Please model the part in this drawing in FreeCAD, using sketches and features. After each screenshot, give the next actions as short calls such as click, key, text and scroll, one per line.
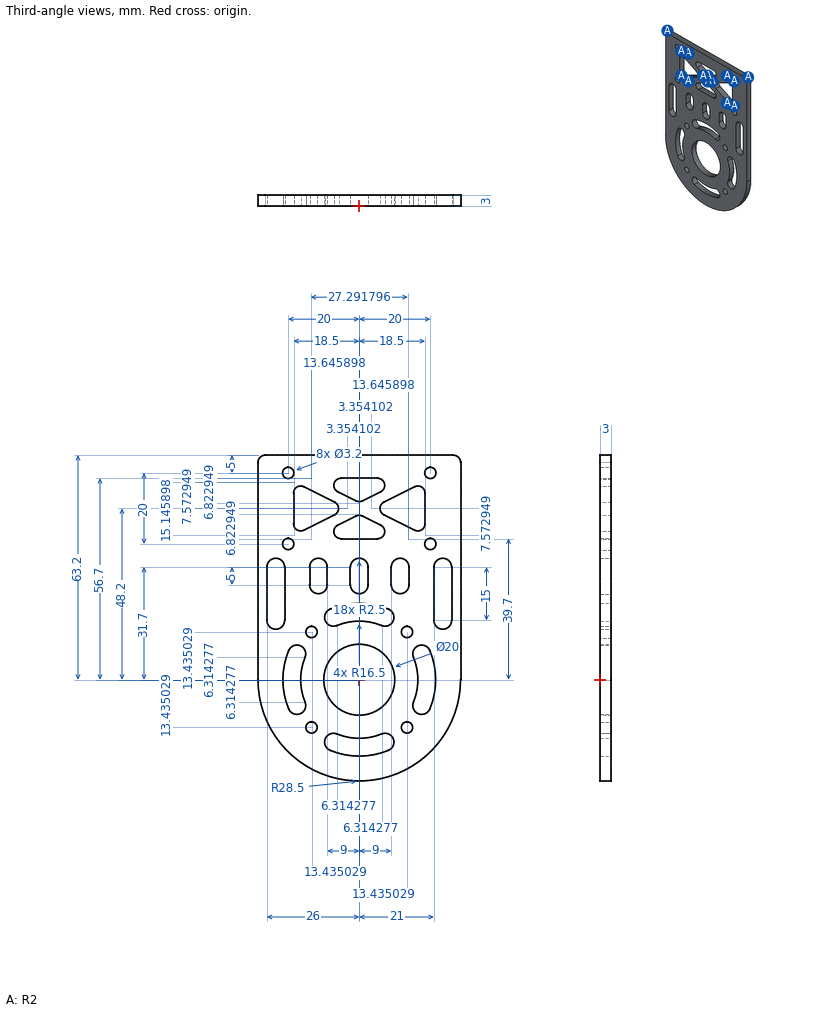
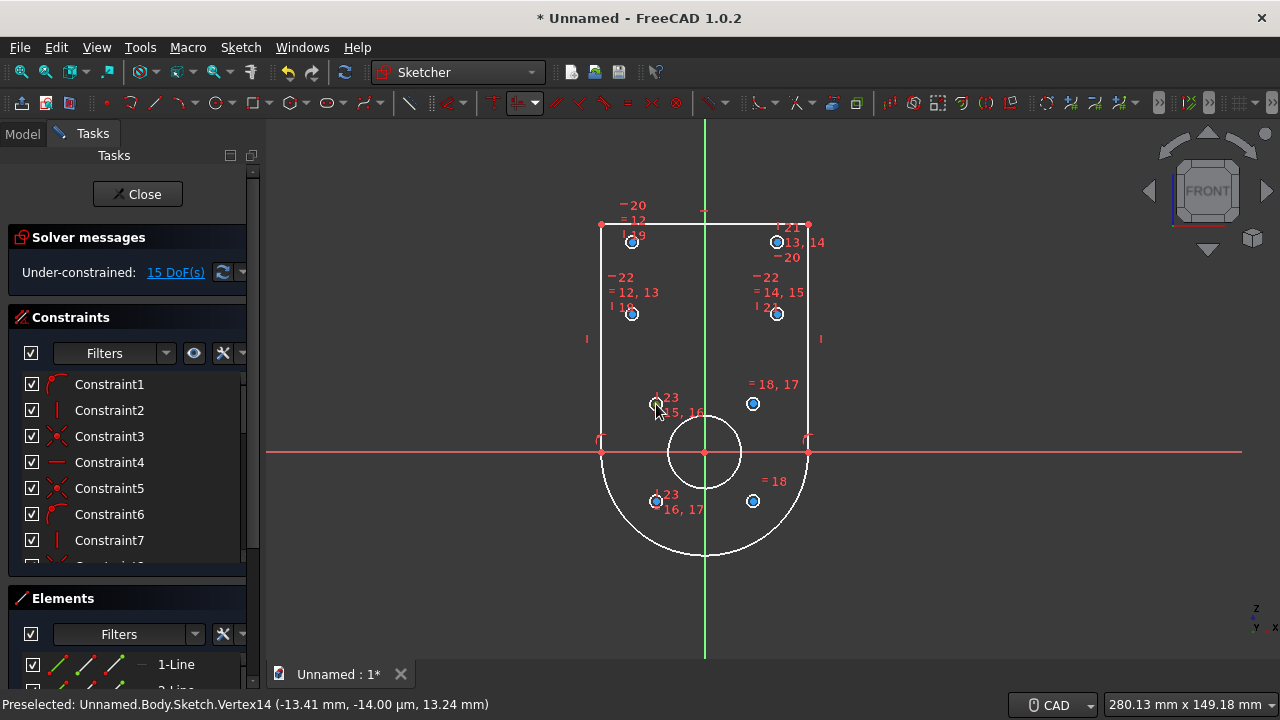
click(753, 404)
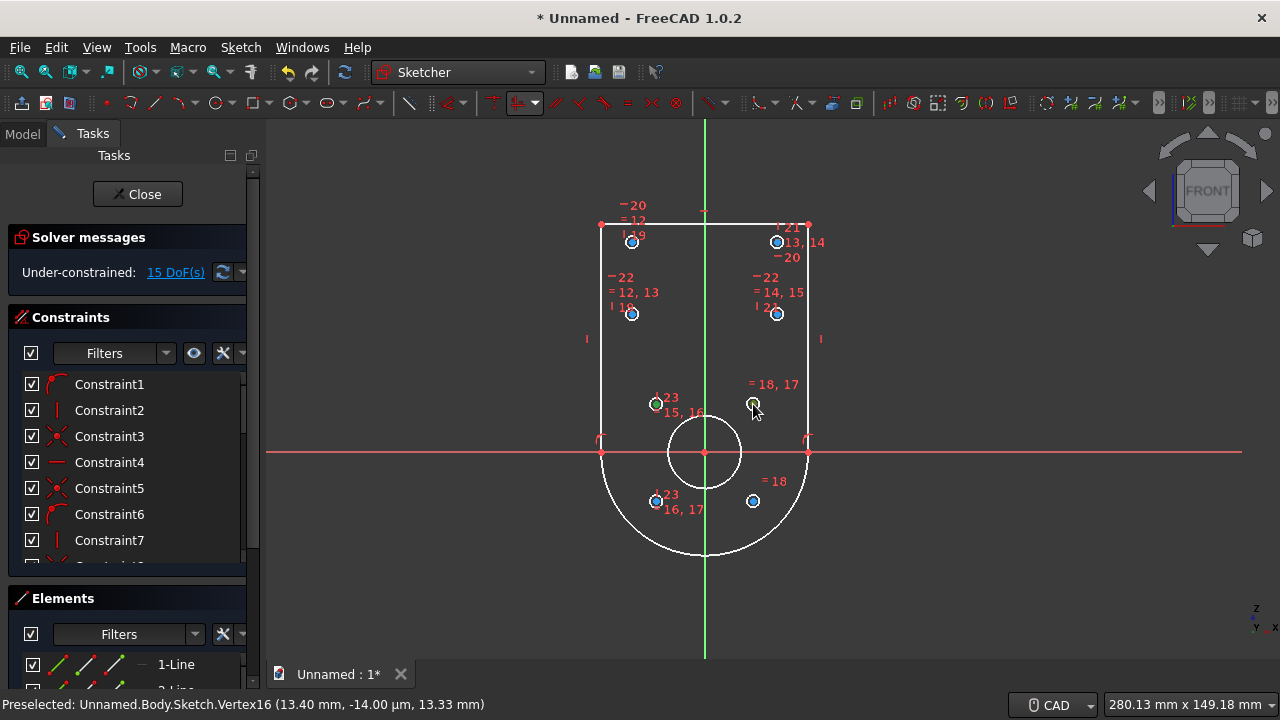
key(h)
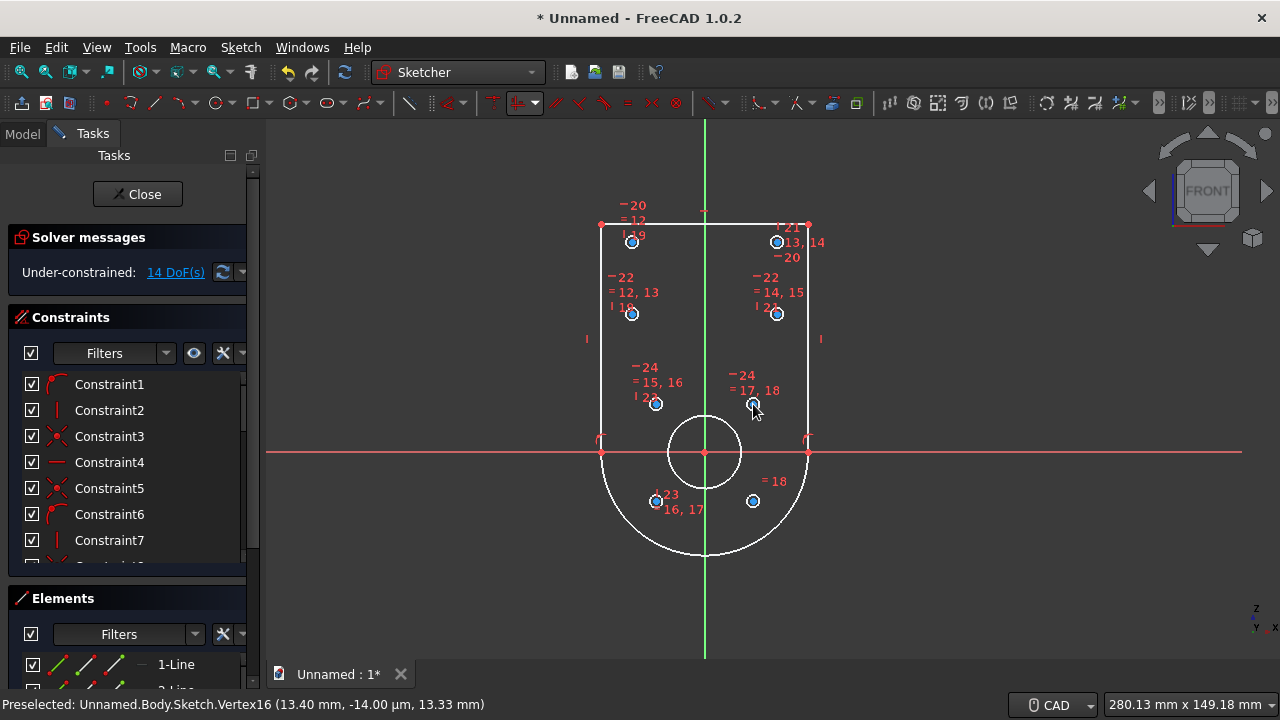
click(753, 404)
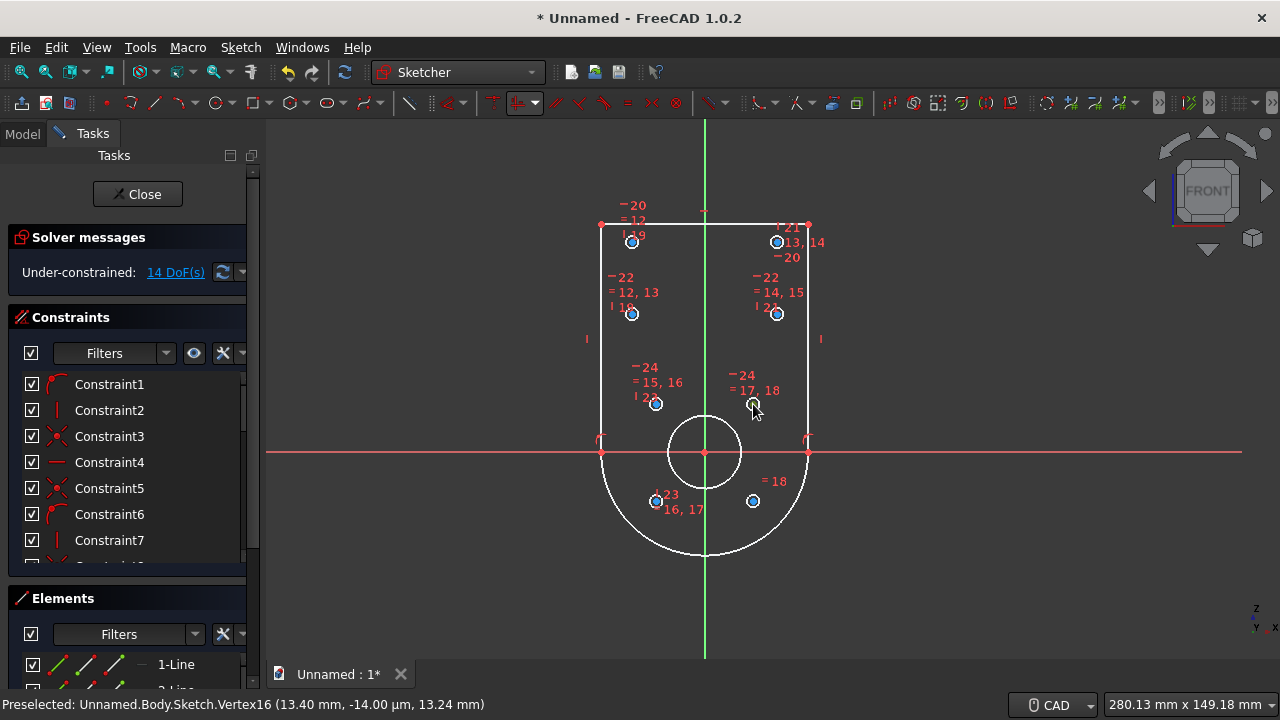
click(753, 501)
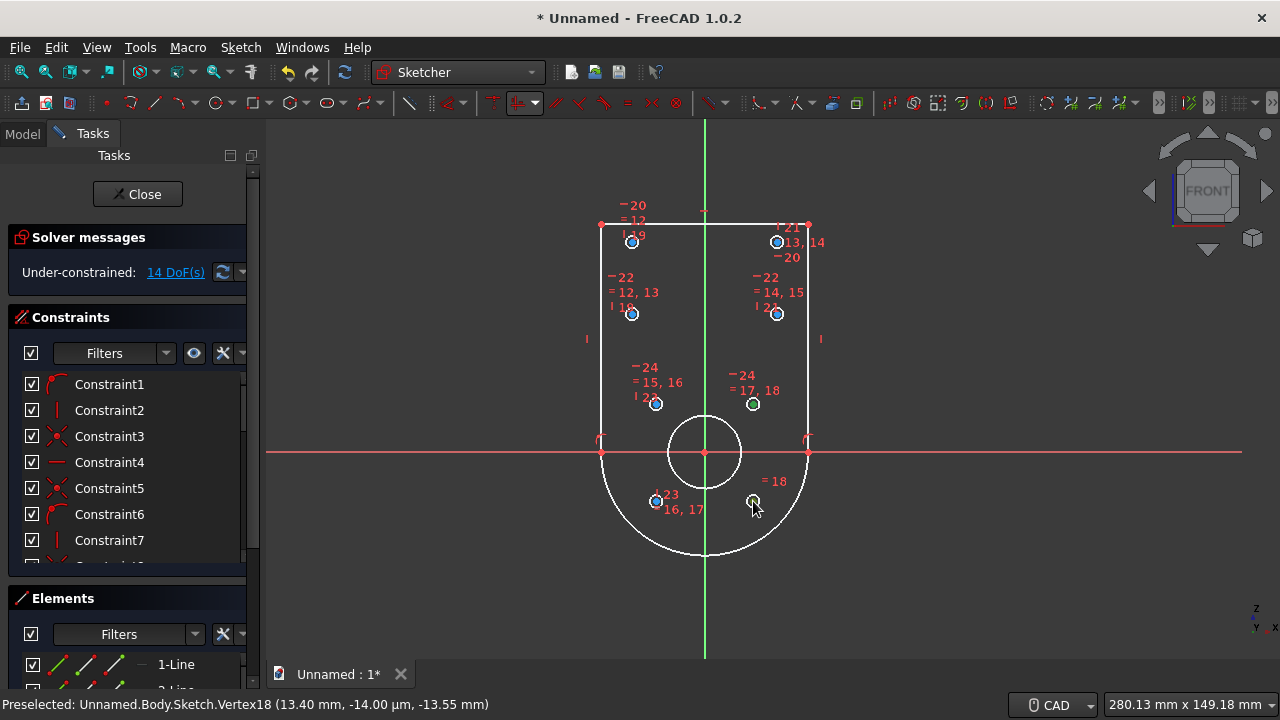
key(v)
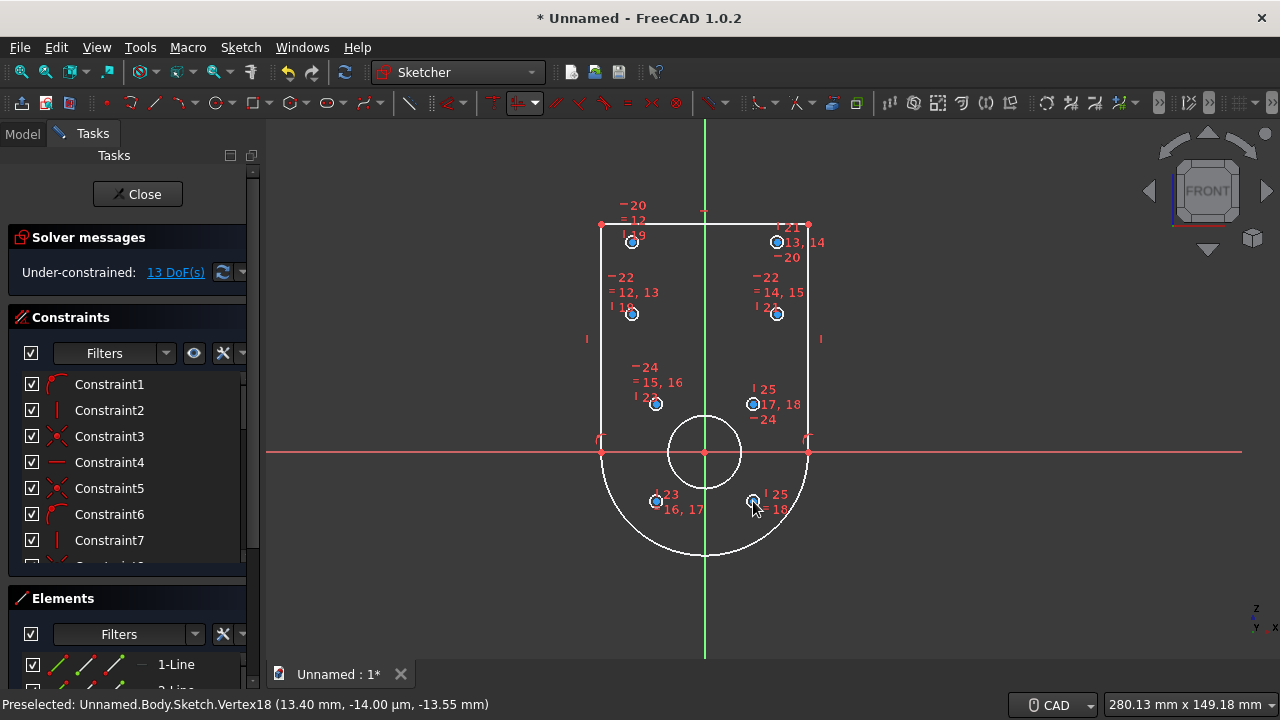
scroll(656, 501, up, 4)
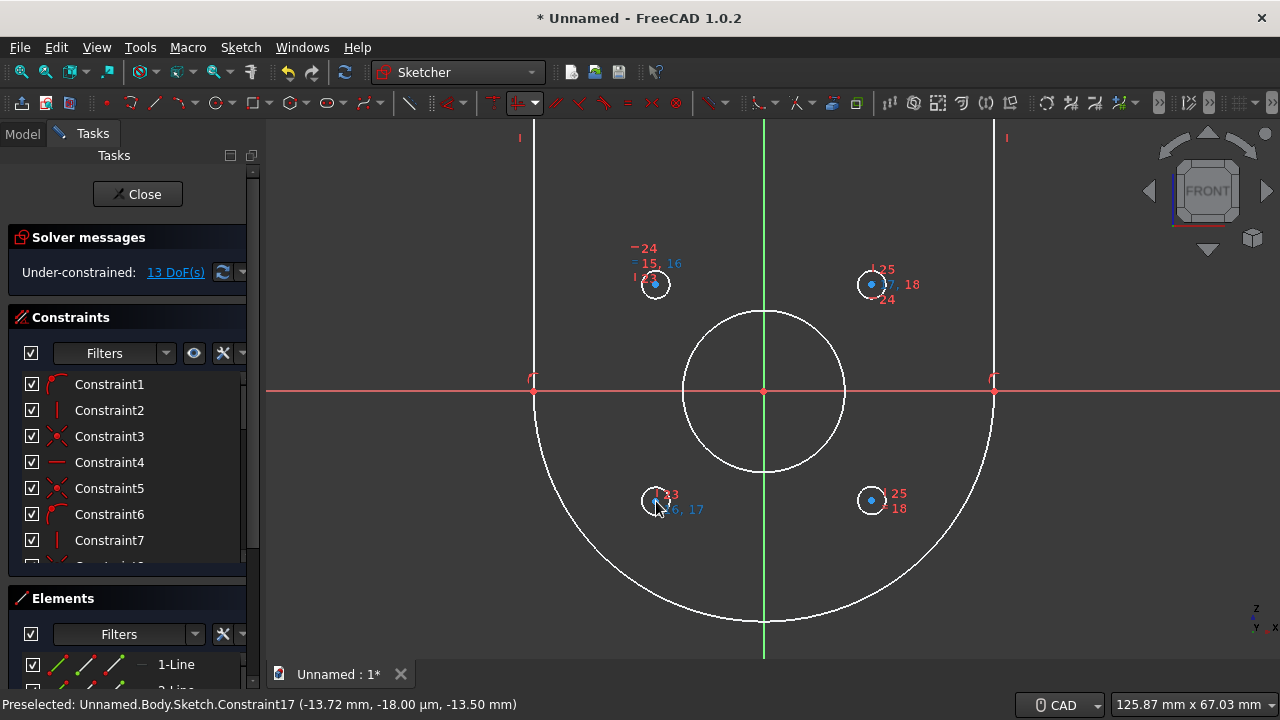
scroll(656, 501, up, 4)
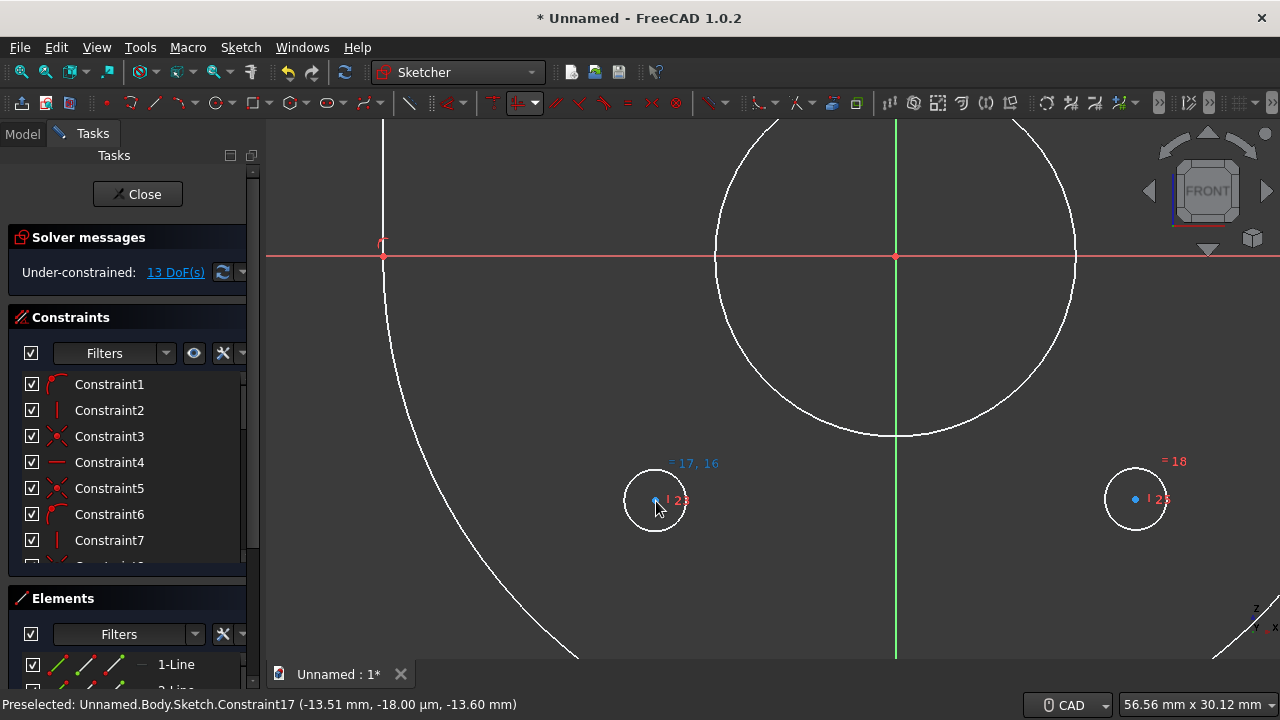
click(655, 501)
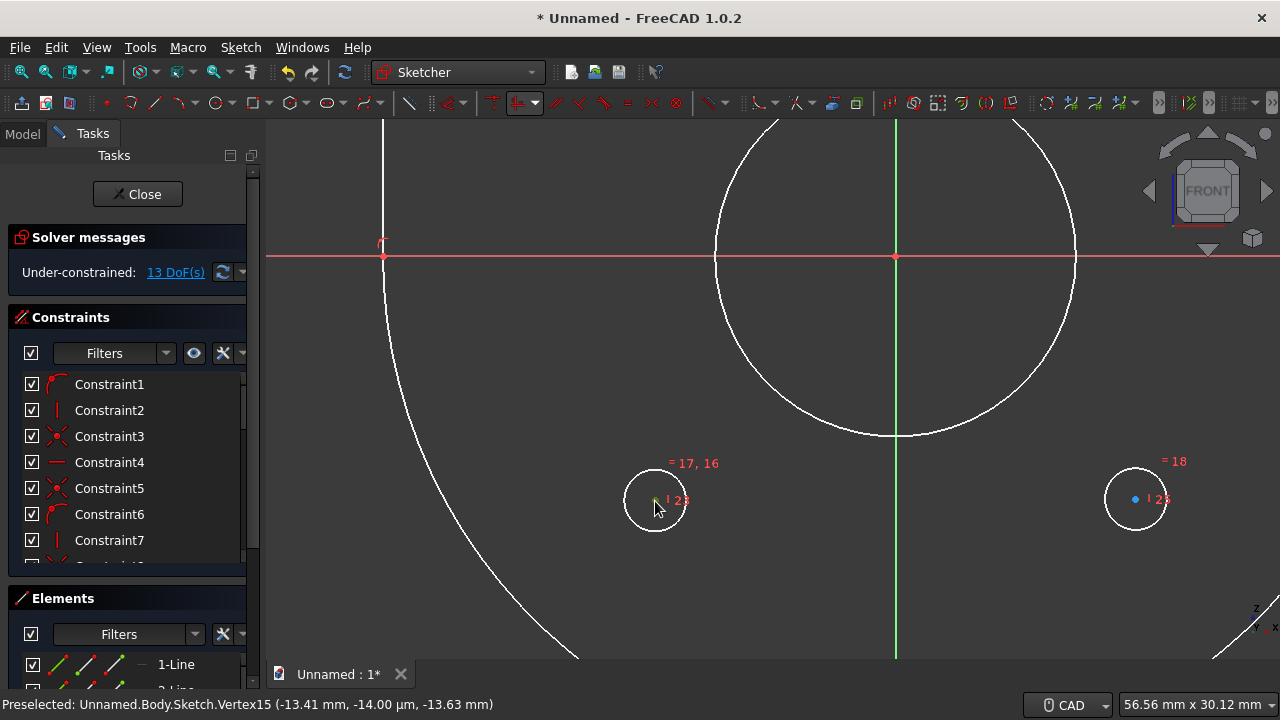
scroll(656, 501, down, 8)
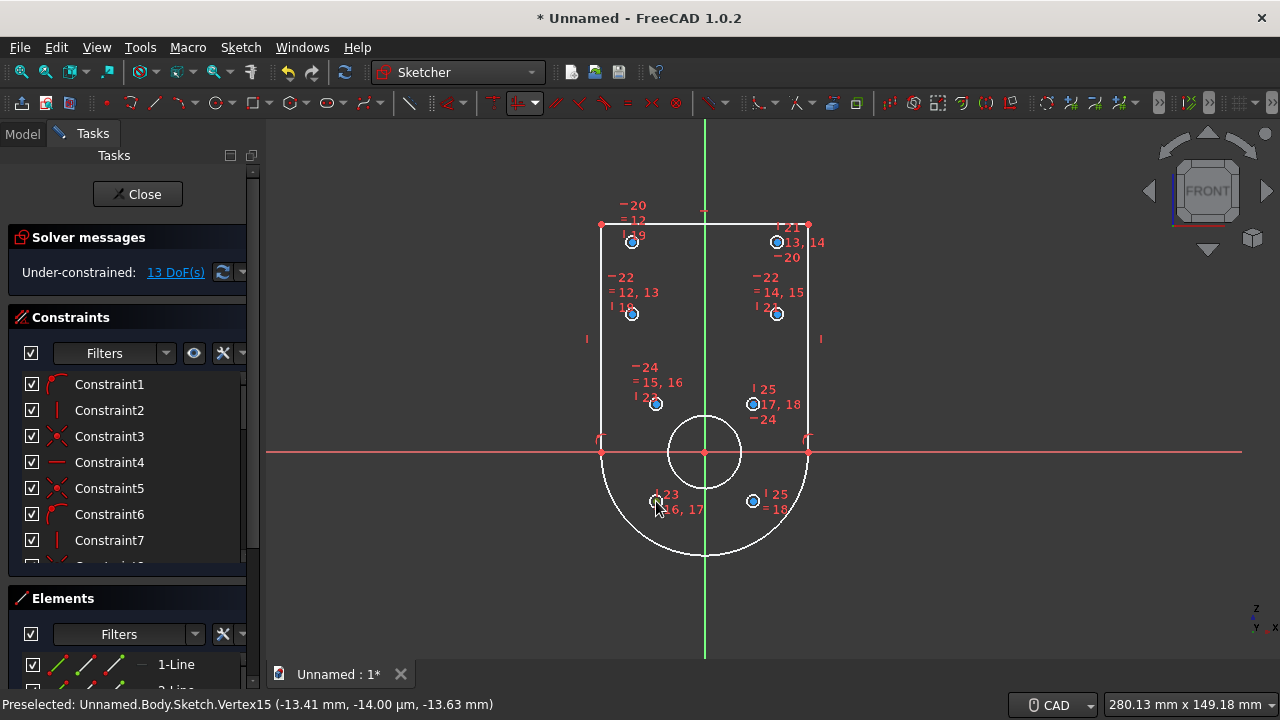
click(753, 501)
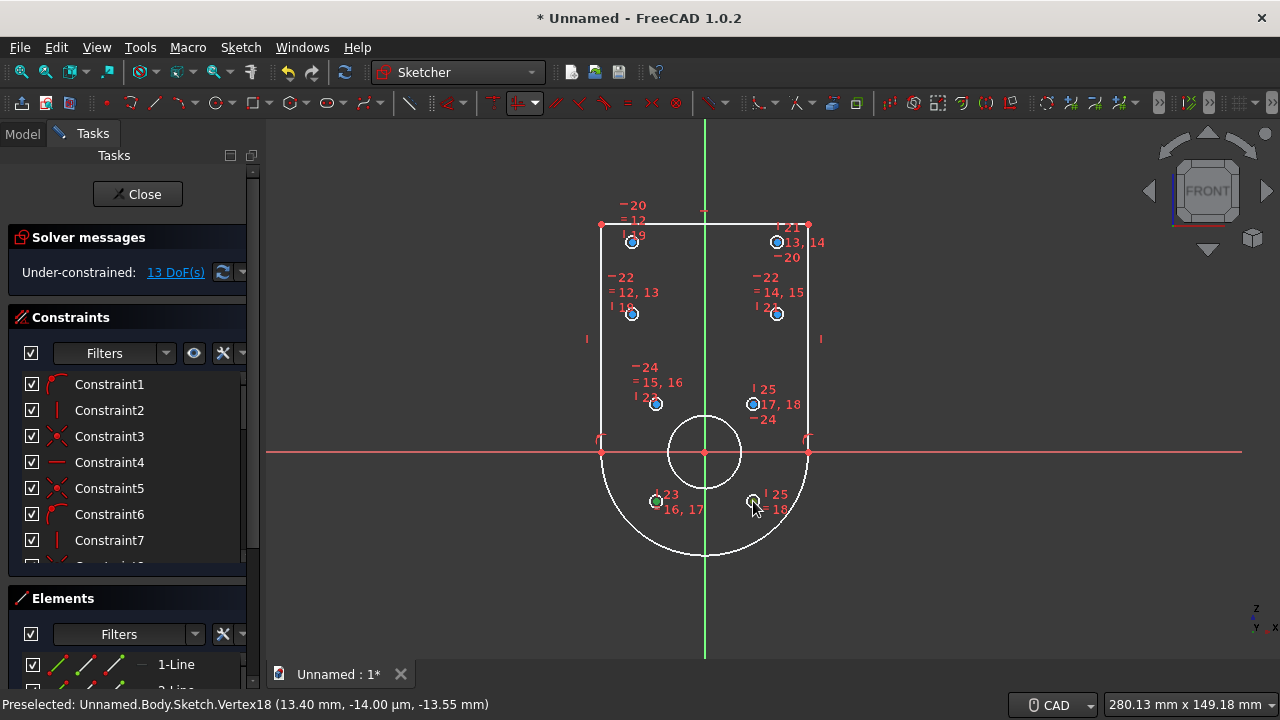
click(538, 104)